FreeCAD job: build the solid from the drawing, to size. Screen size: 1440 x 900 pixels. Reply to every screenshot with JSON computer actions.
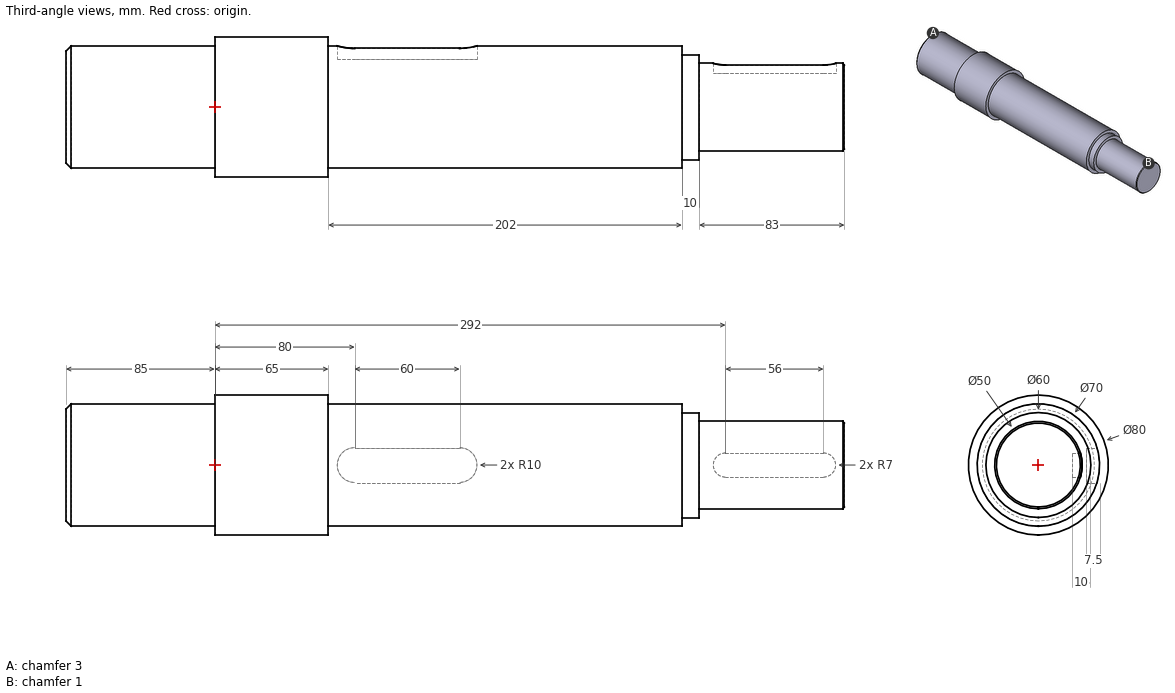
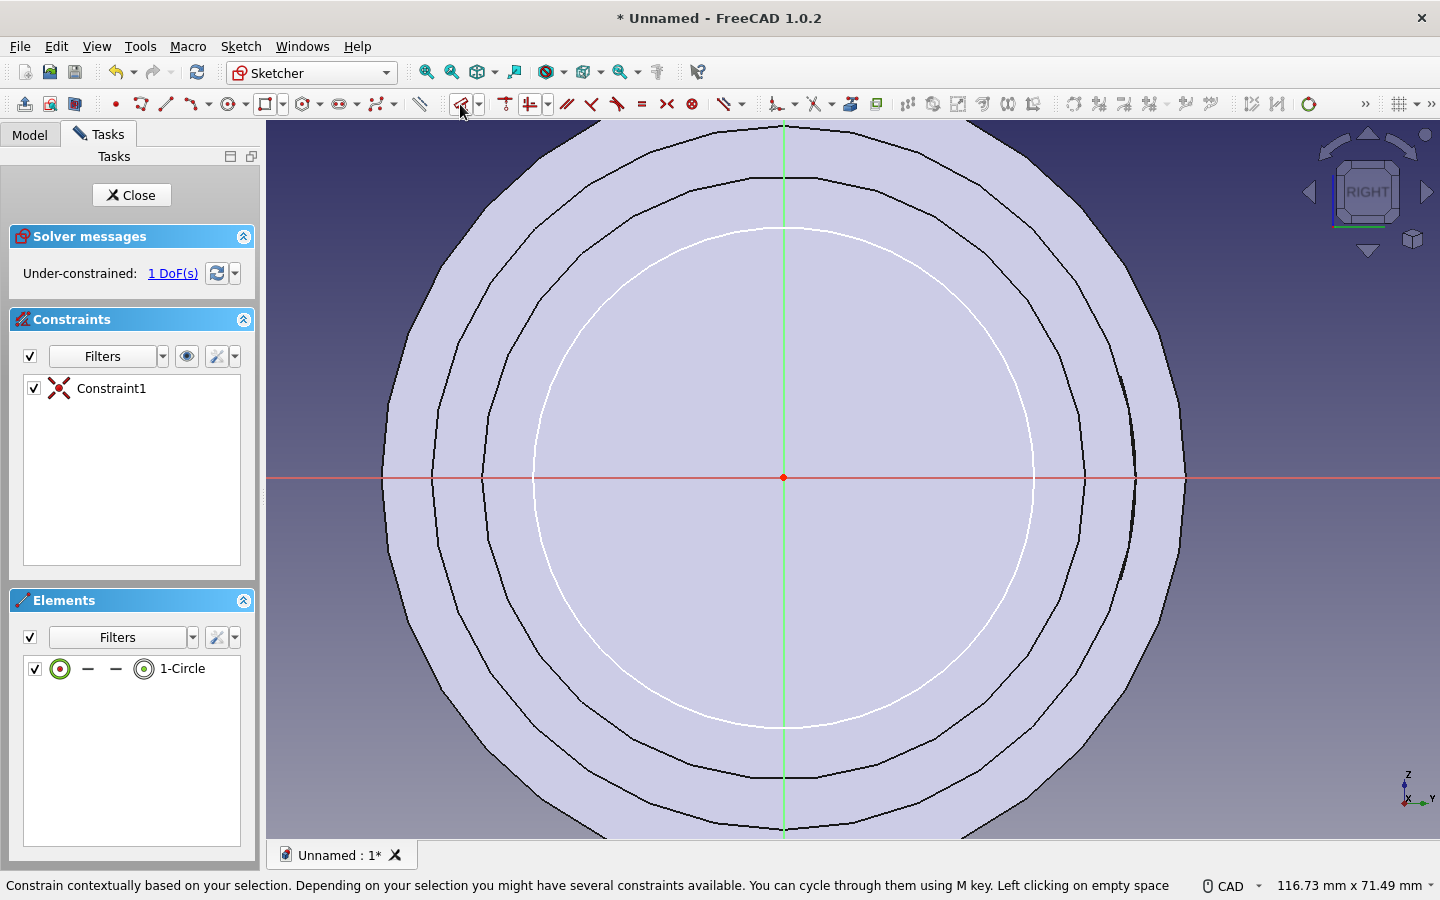
{"action": "left_click", "coordinate": [960, 300]}
{"action": "left_click", "coordinate": [983, 277]}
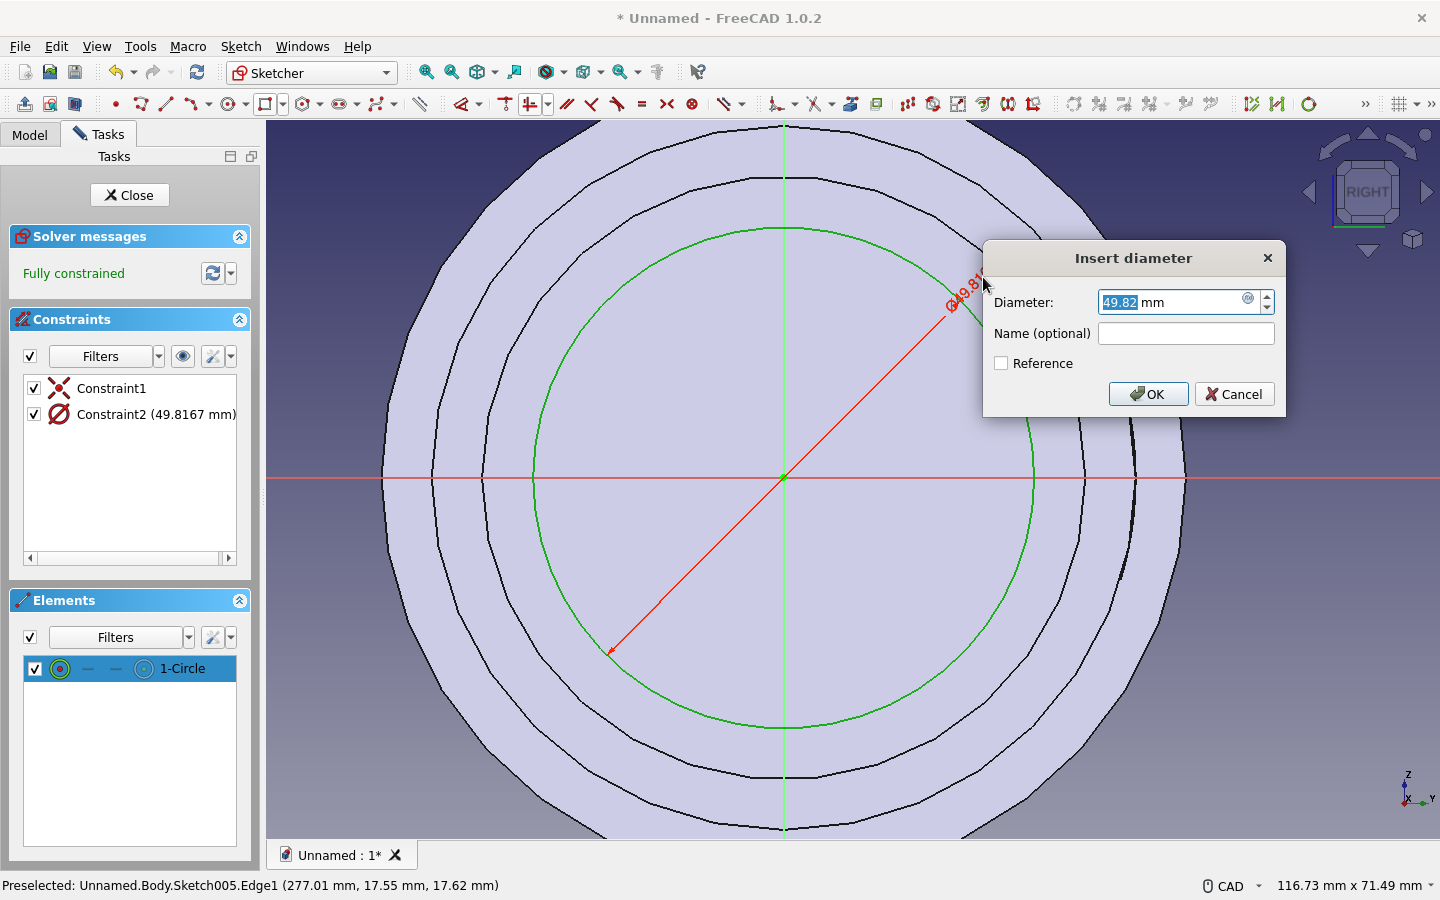
{"action": "type", "text": "50"}
{"action": "key", "text": "Return"}
{"action": "key", "text": "Escape"}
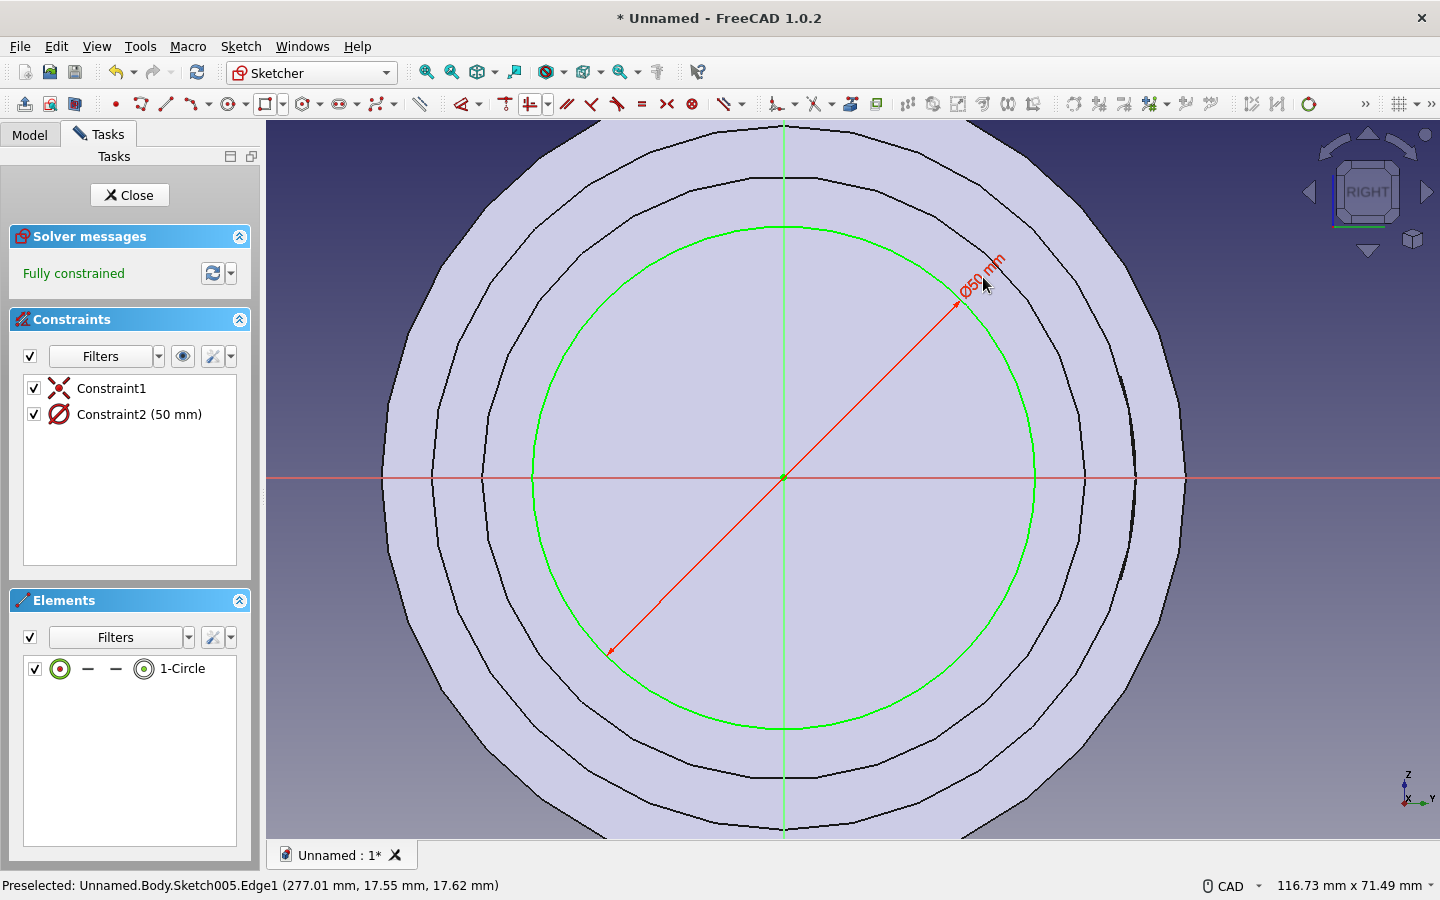
{"action": "left_click", "coordinate": [130, 195]}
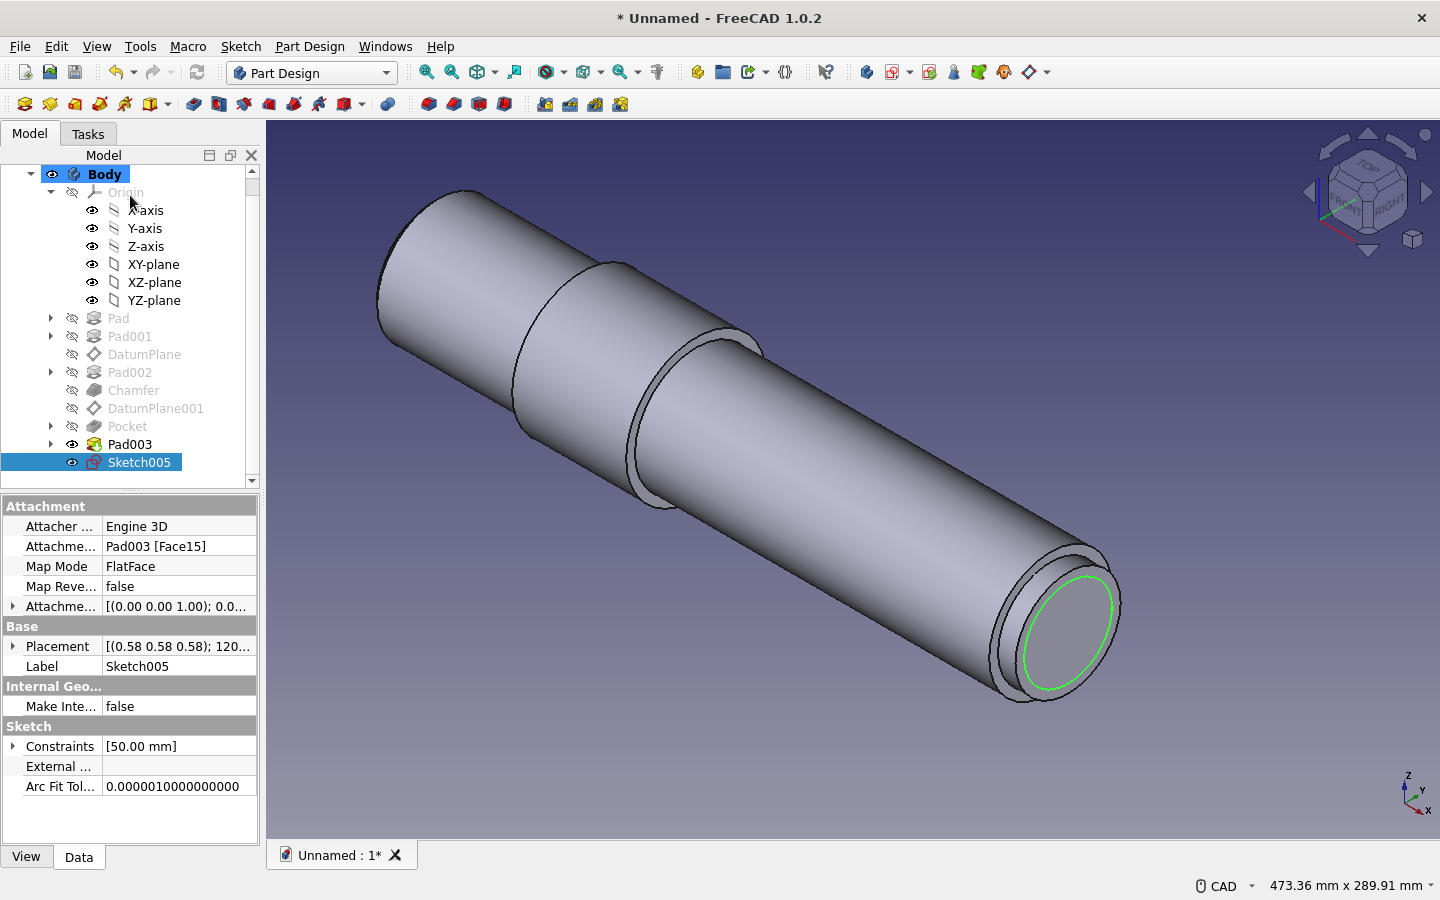
{"action": "left_click", "coordinate": [25, 104]}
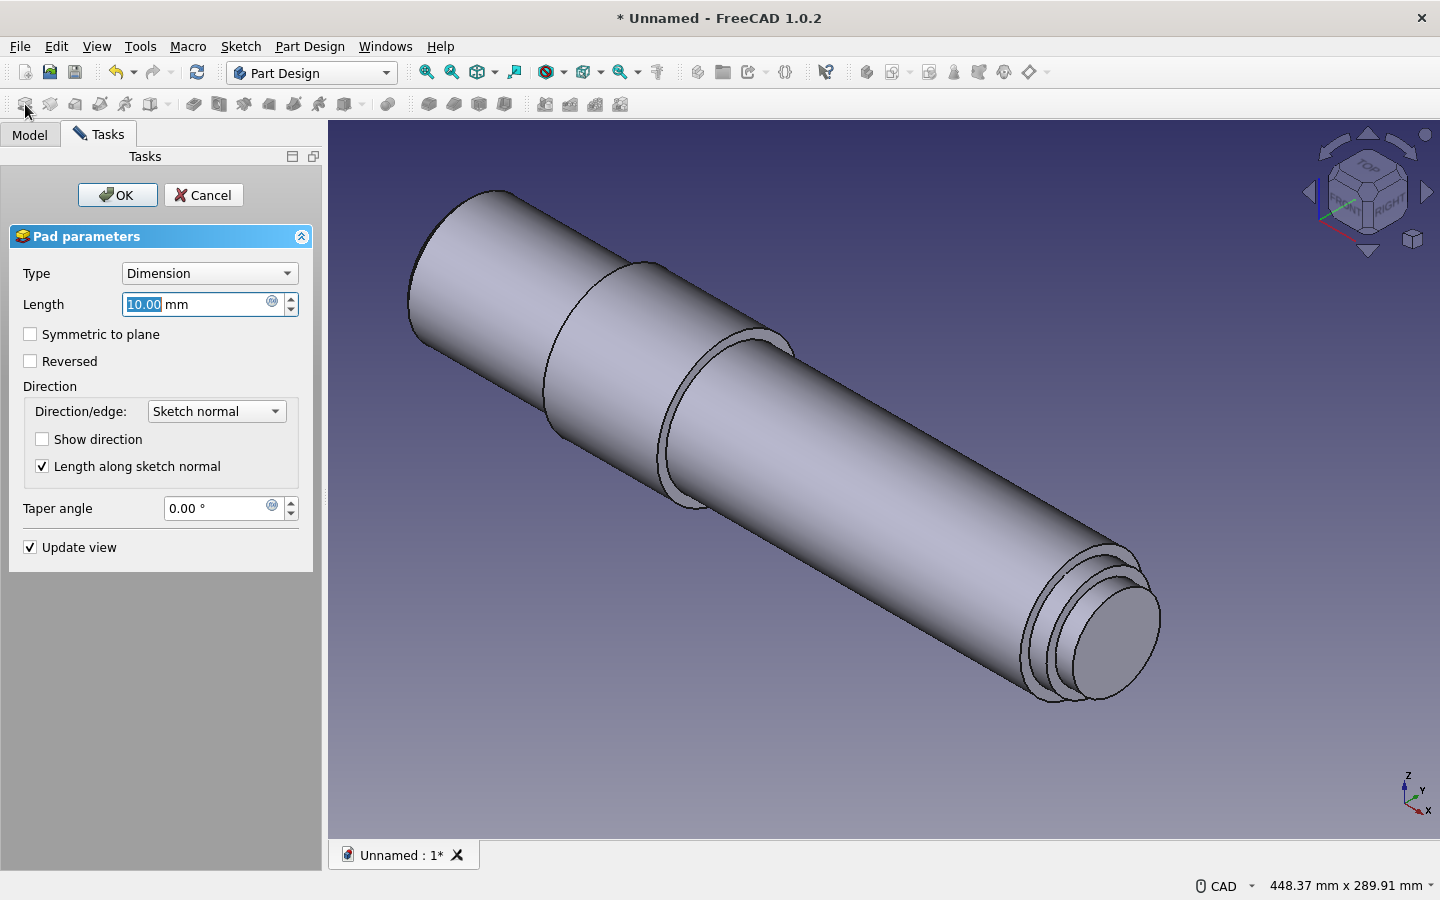
{"action": "type", "text": "83"}
{"action": "key", "text": "Tab"}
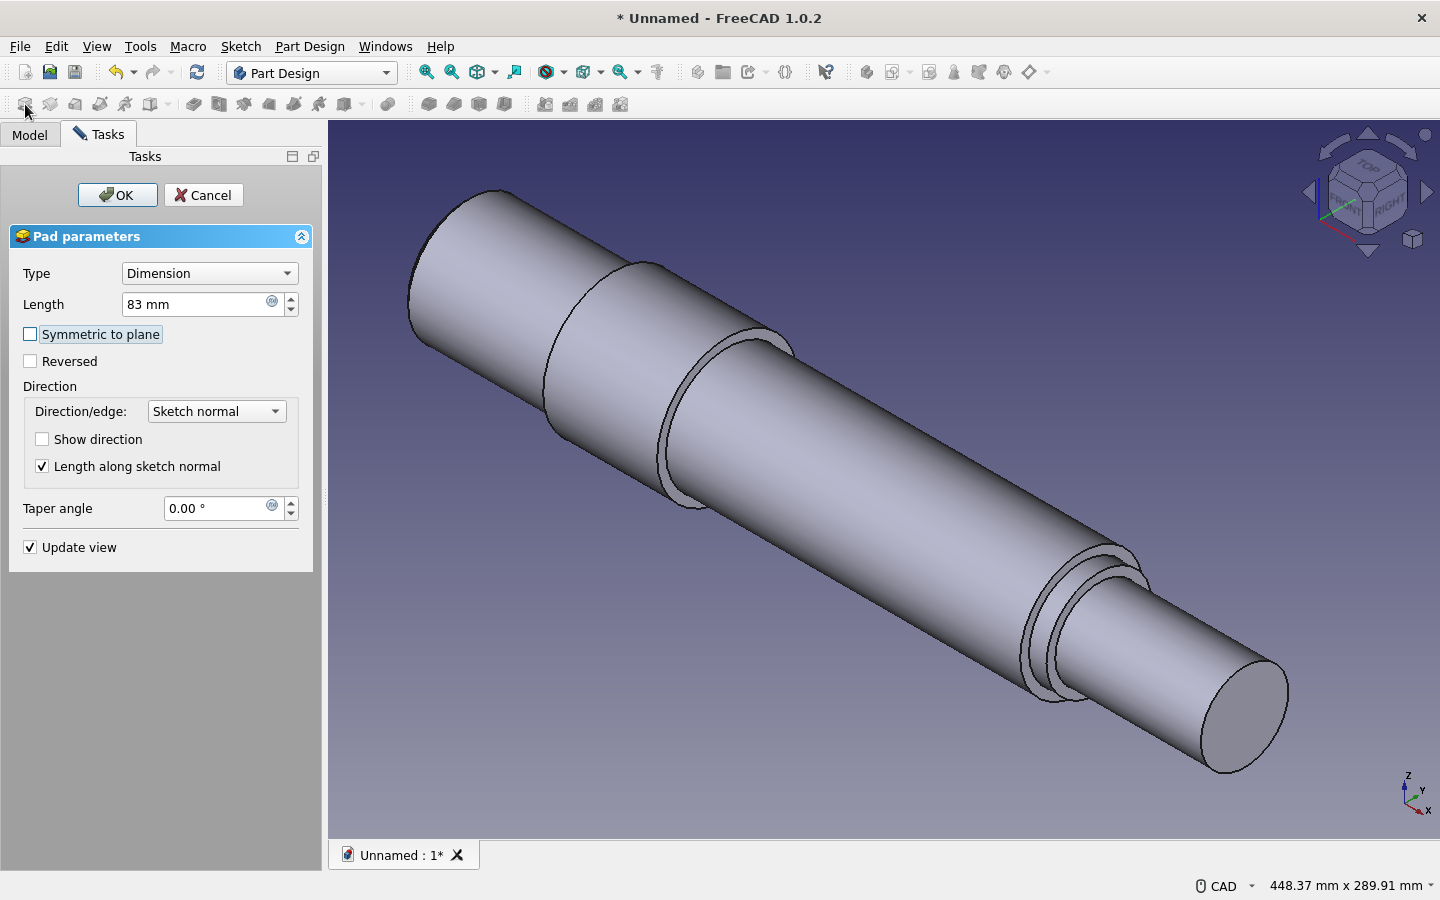
{"action": "left_click", "coordinate": [118, 195]}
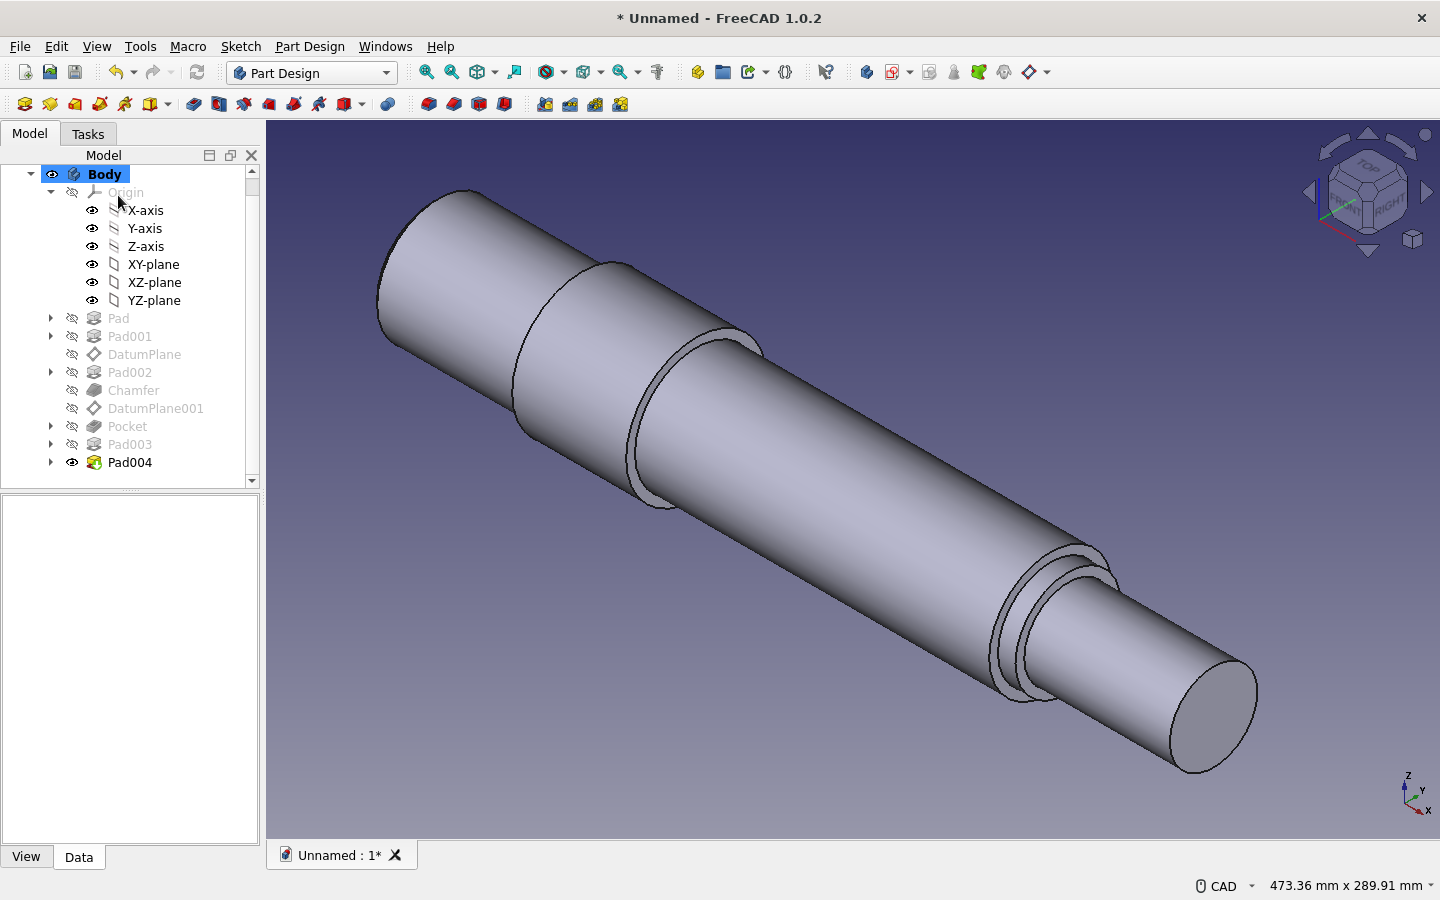
{"action": "left_click", "coordinate": [137, 282]}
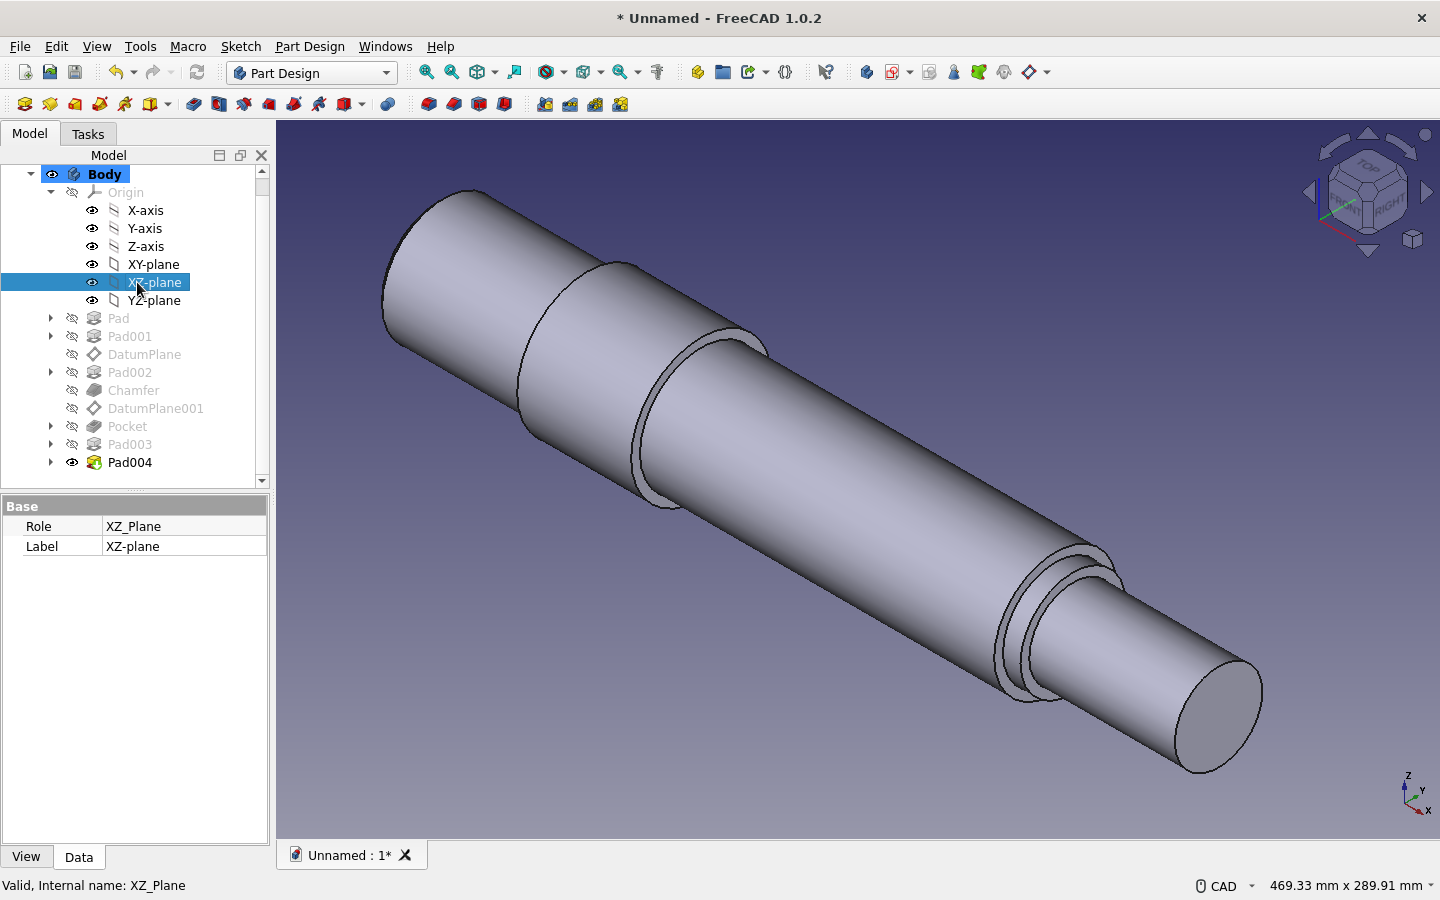
{"action": "left_click", "coordinate": [1028, 72]}